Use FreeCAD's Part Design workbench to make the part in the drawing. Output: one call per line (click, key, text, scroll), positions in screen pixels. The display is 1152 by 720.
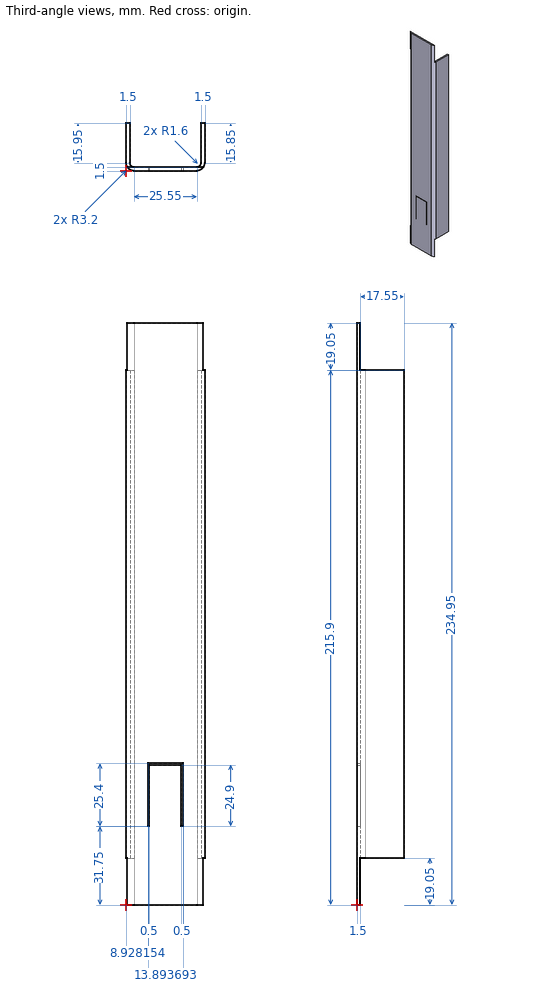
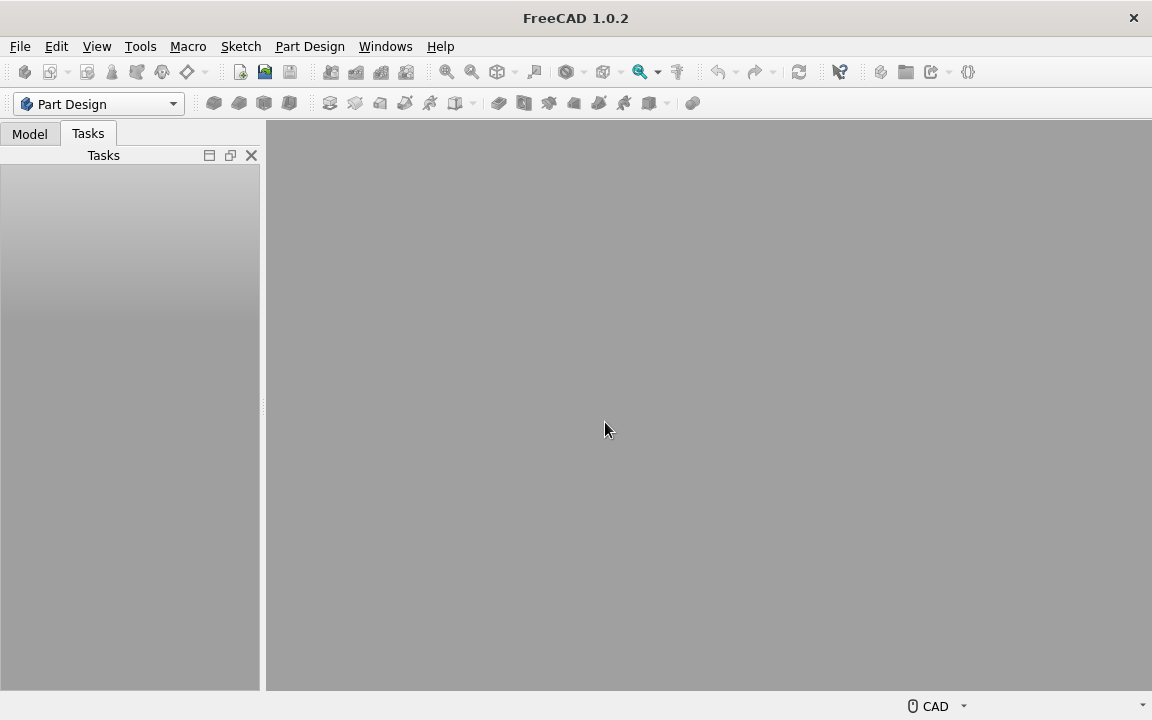
click(240, 72)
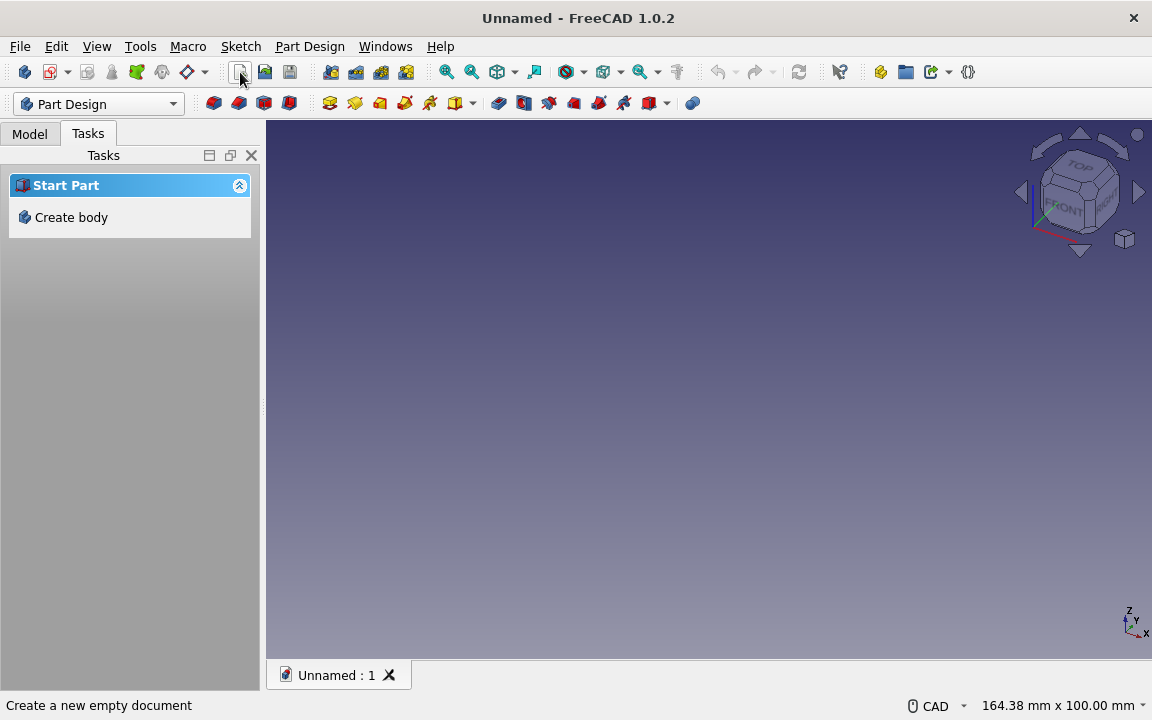
click(50, 72)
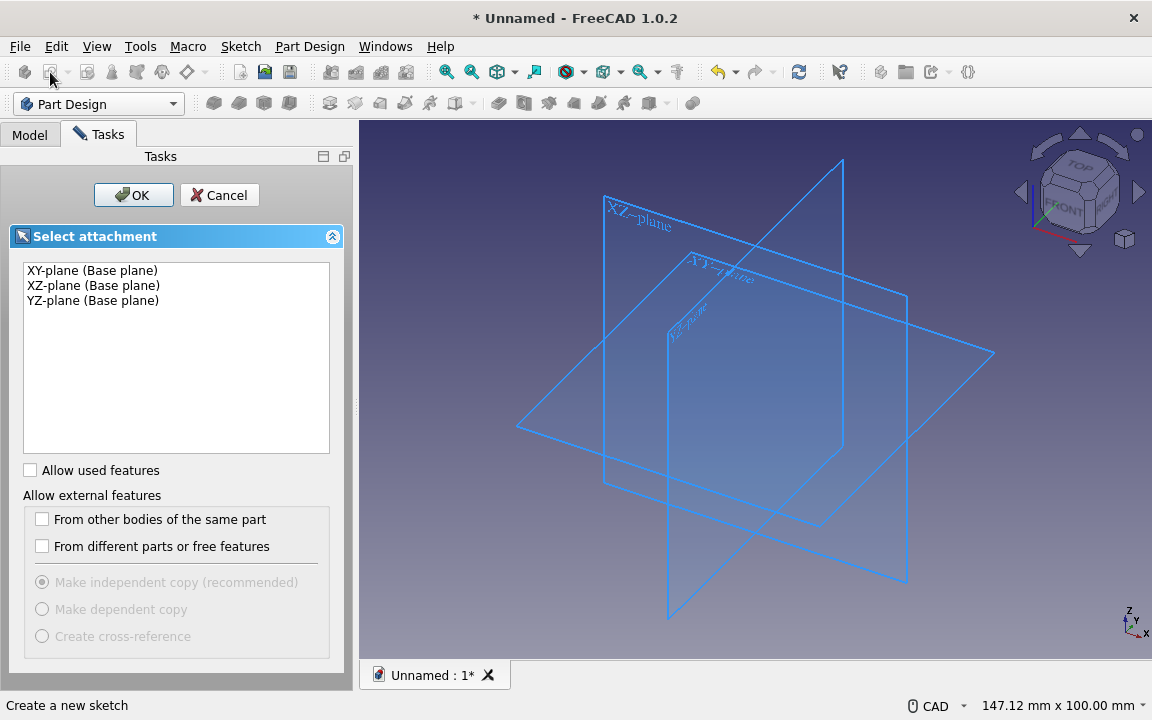
click(84, 270)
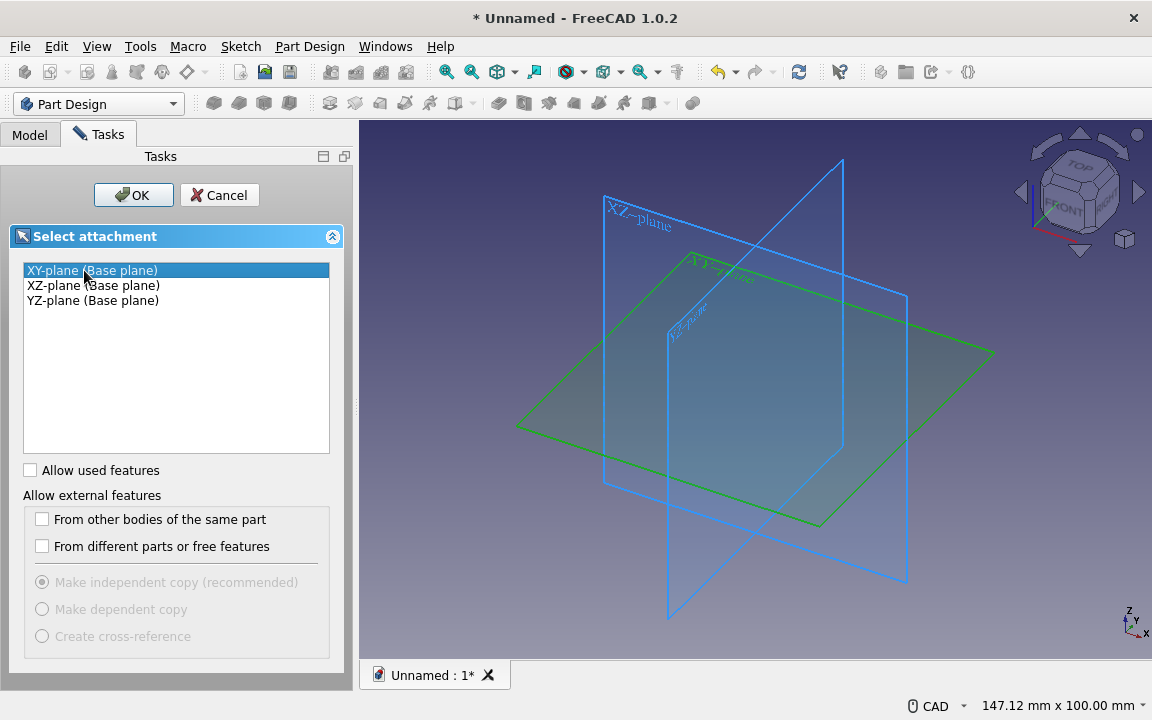
click(134, 195)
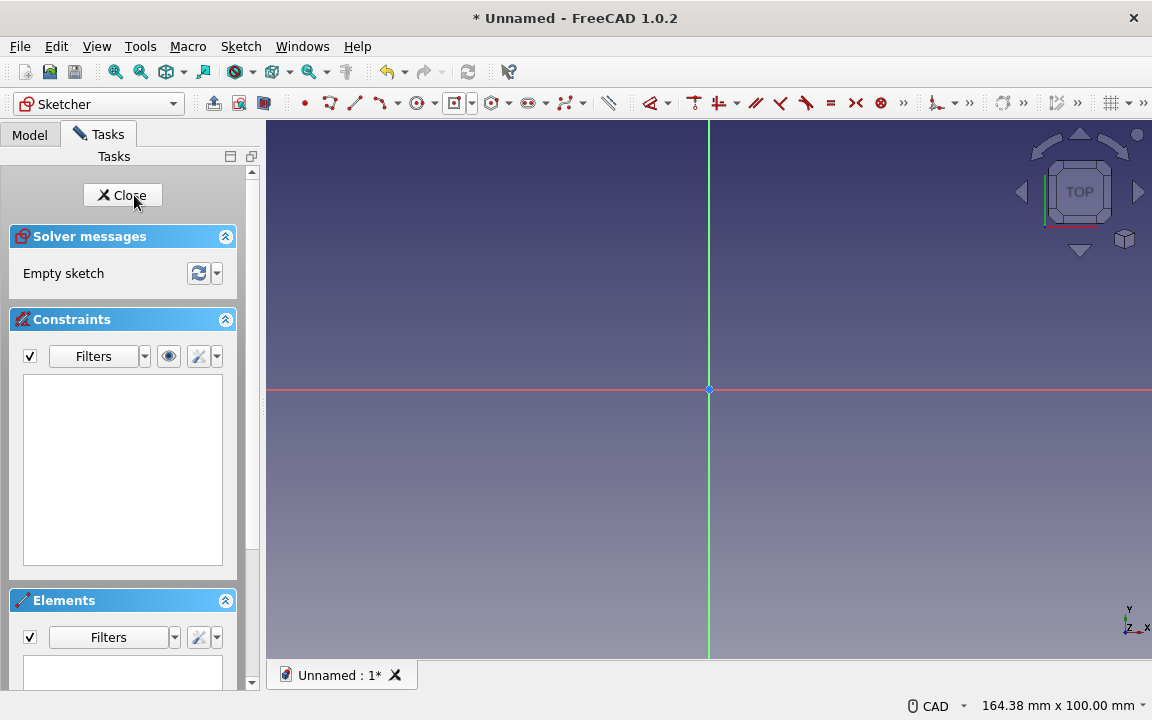
scroll(884, 308, up, 5)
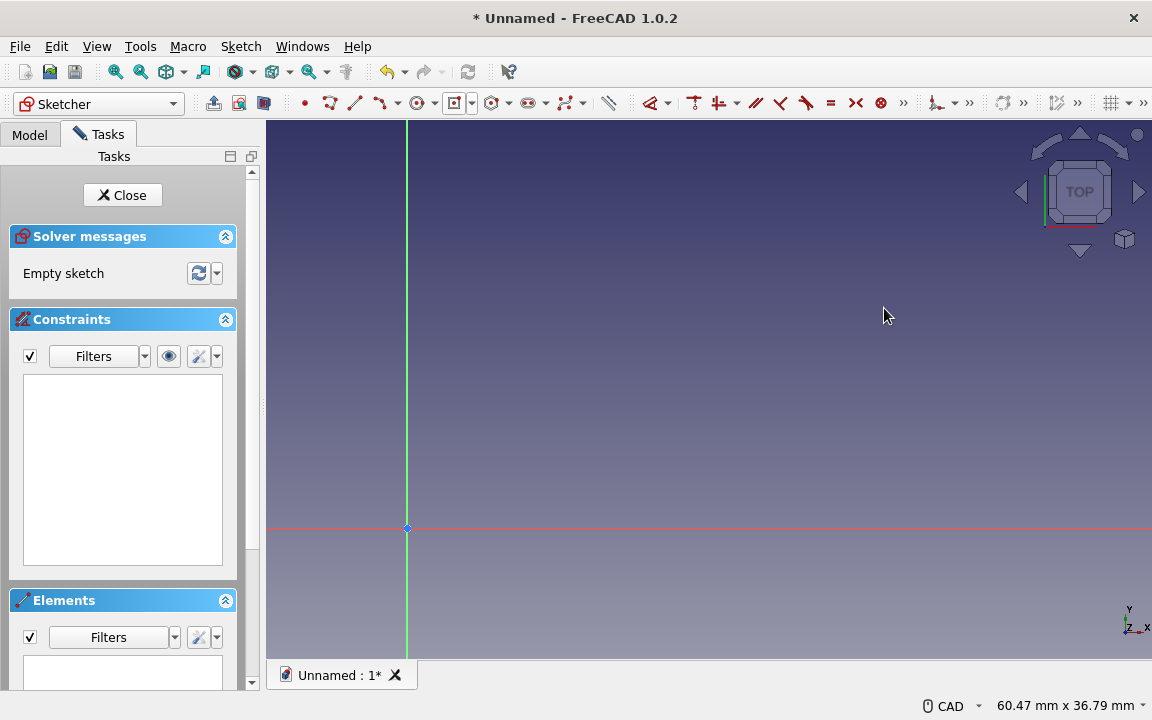
click(355, 104)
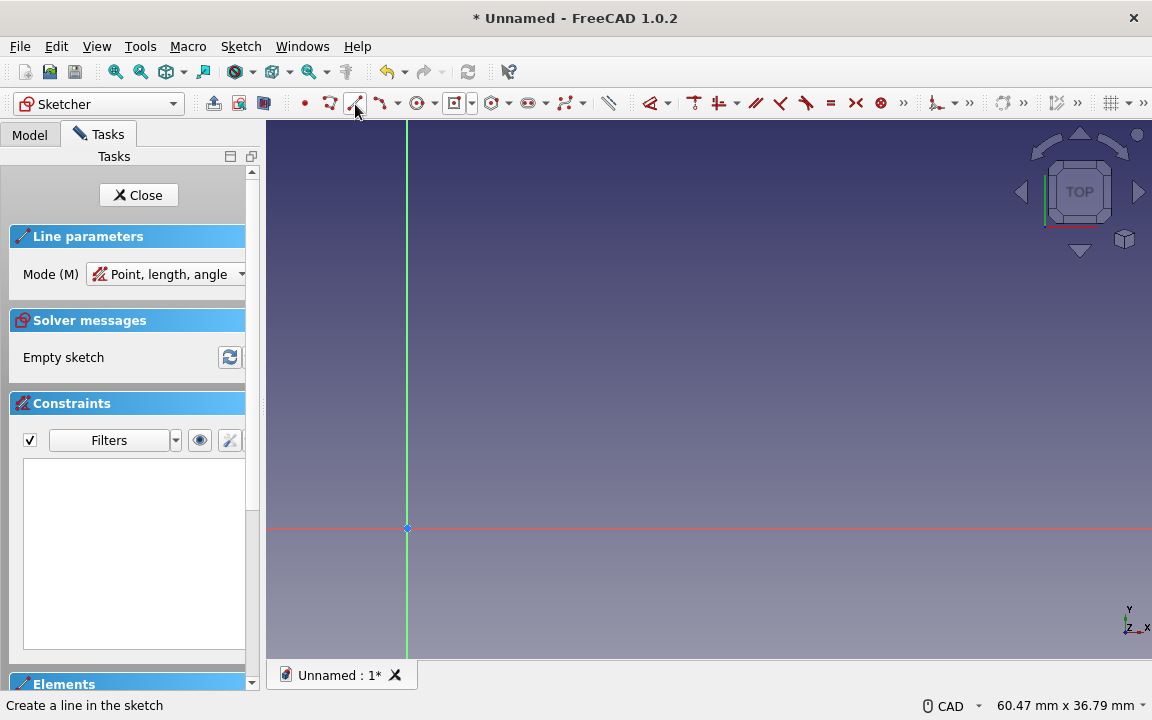
click(827, 507)
click(453, 507)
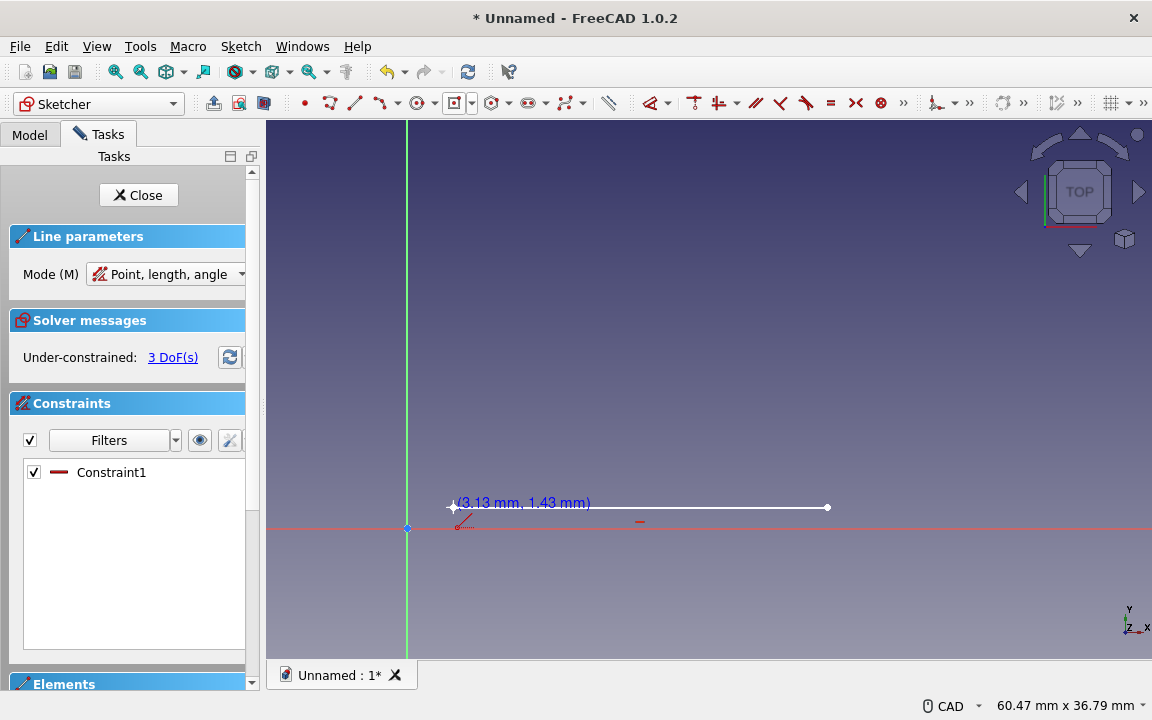
click(330, 104)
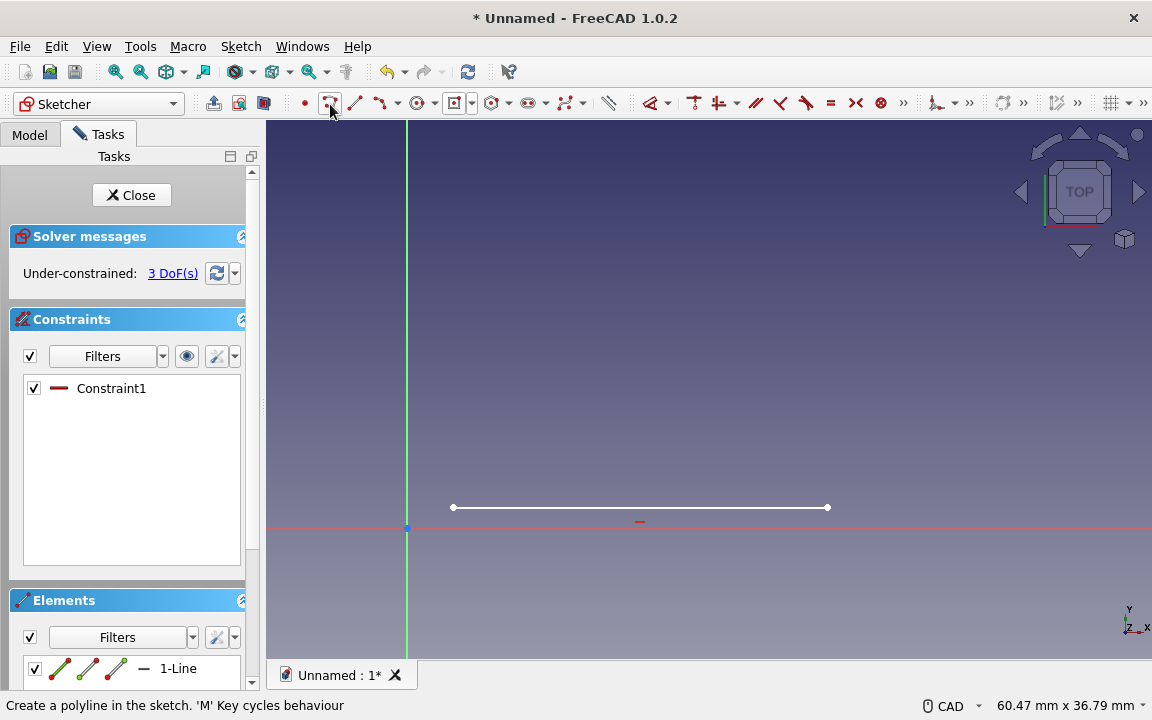
click(429, 484)
click(429, 250)
click(407, 250)
click(416, 482)
right_click(416, 482)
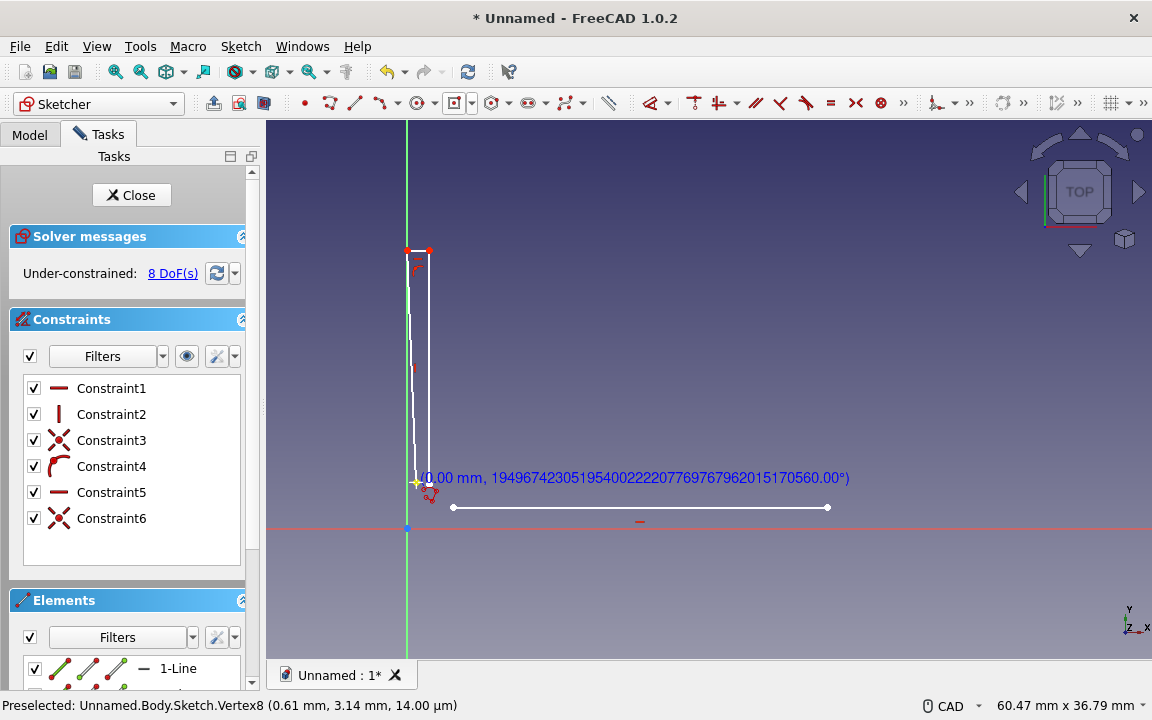
key(g)
key(l)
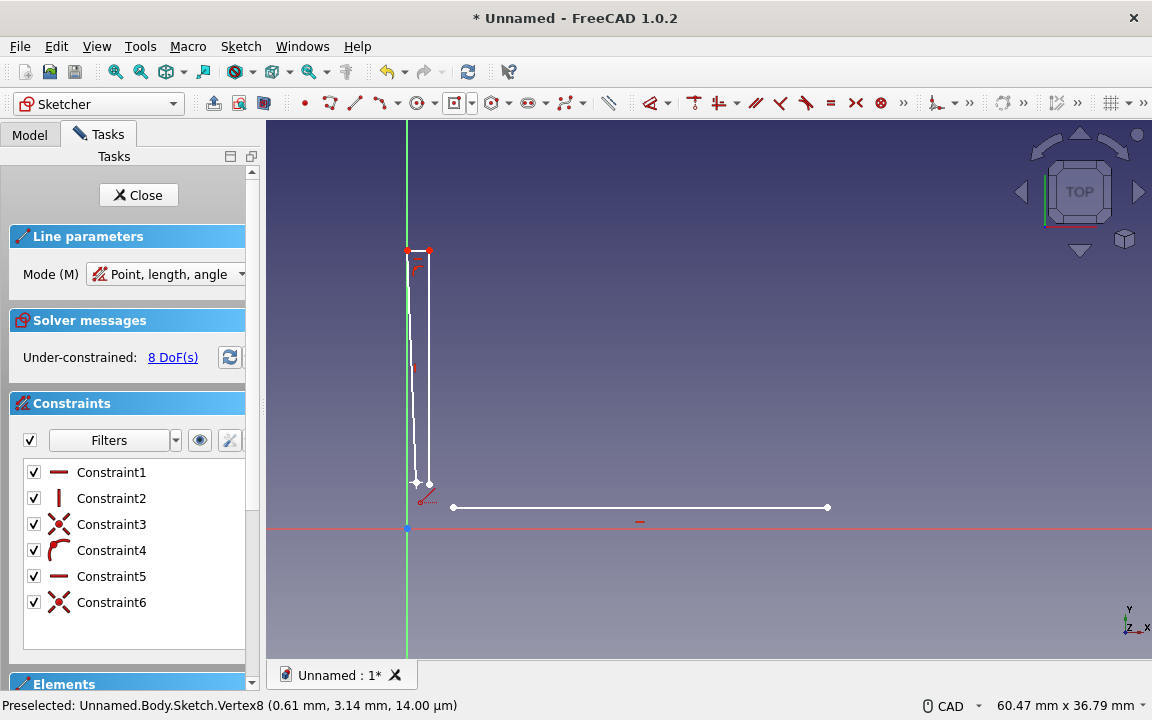
click(454, 529)
click(825, 520)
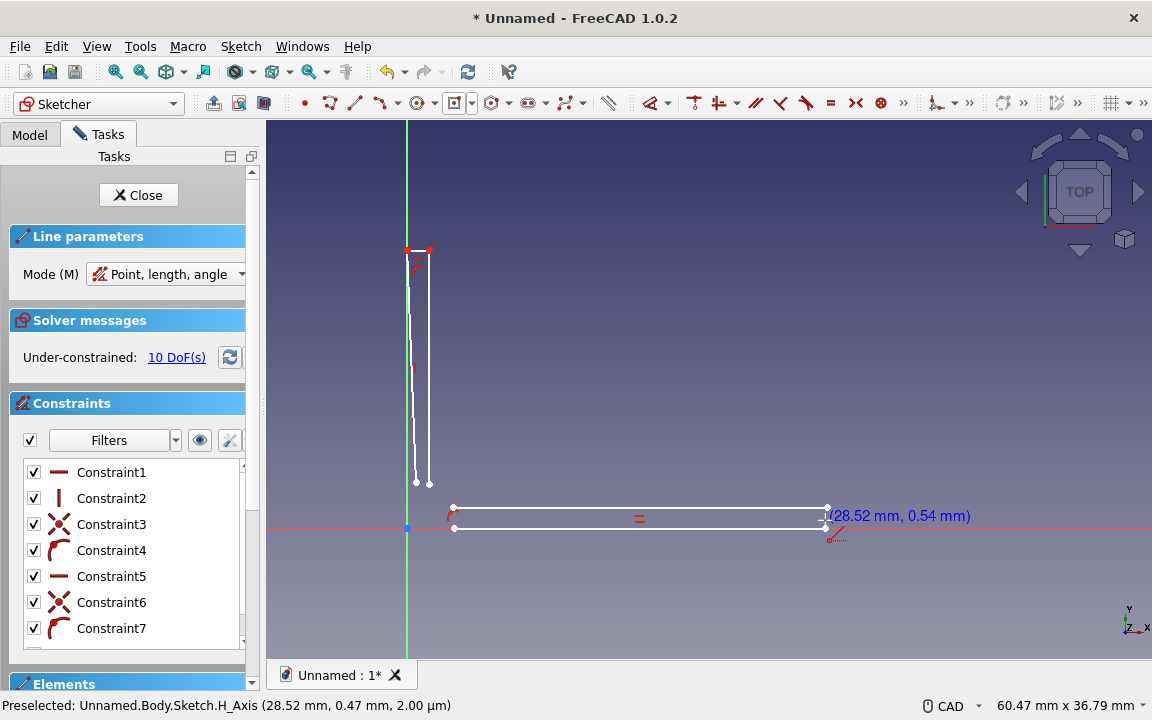
click(330, 104)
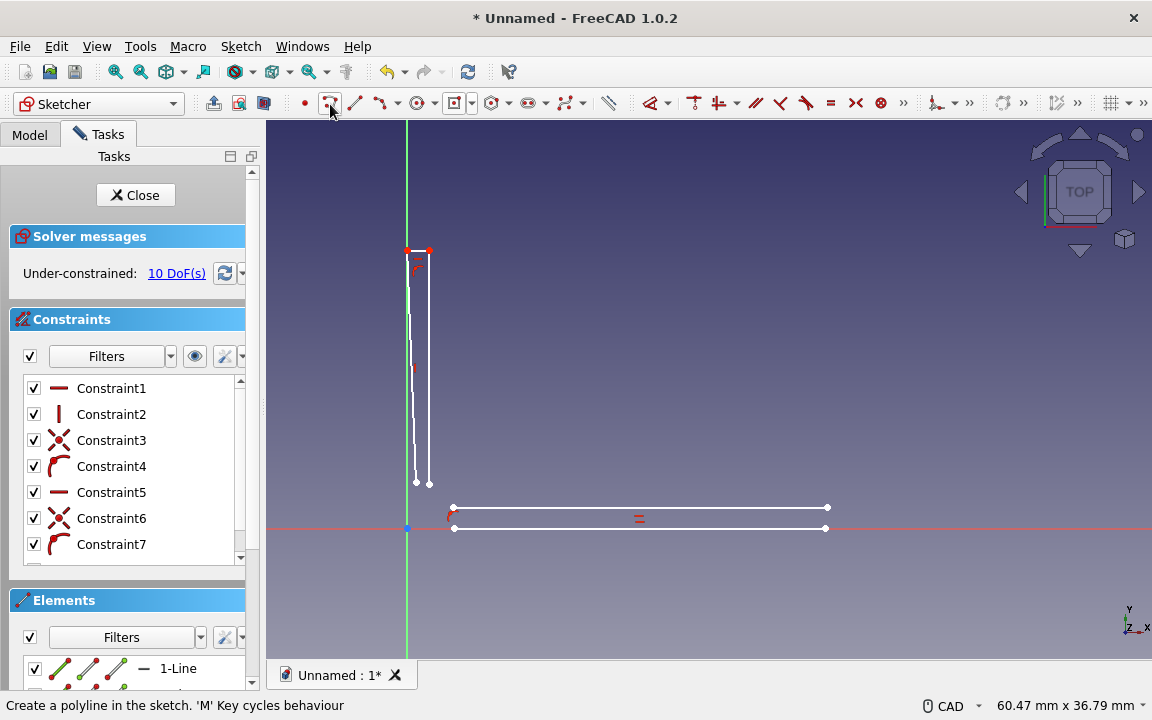
click(872, 482)
click(872, 250)
click(850, 250)
click(850, 484)
right_click(850, 484)